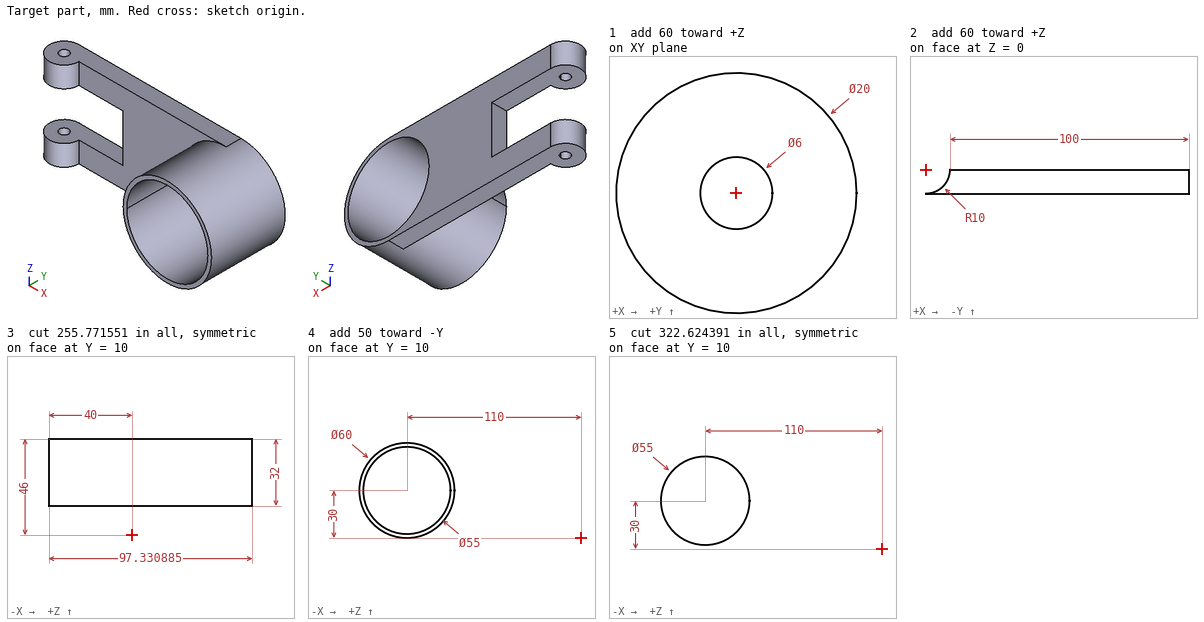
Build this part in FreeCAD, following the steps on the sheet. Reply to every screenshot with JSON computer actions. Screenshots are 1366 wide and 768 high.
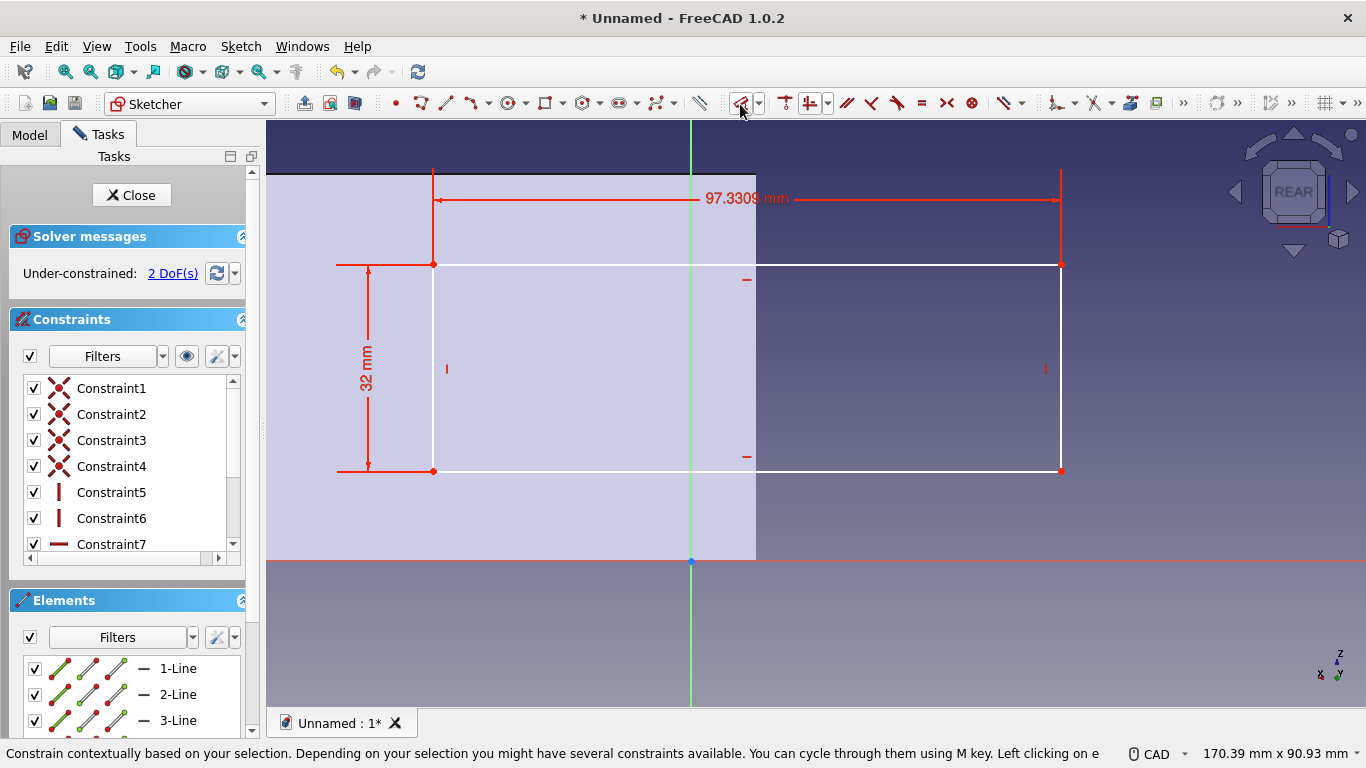
{"action": "left_click", "coordinate": [433, 265]}
{"action": "left_click", "coordinate": [562, 595]}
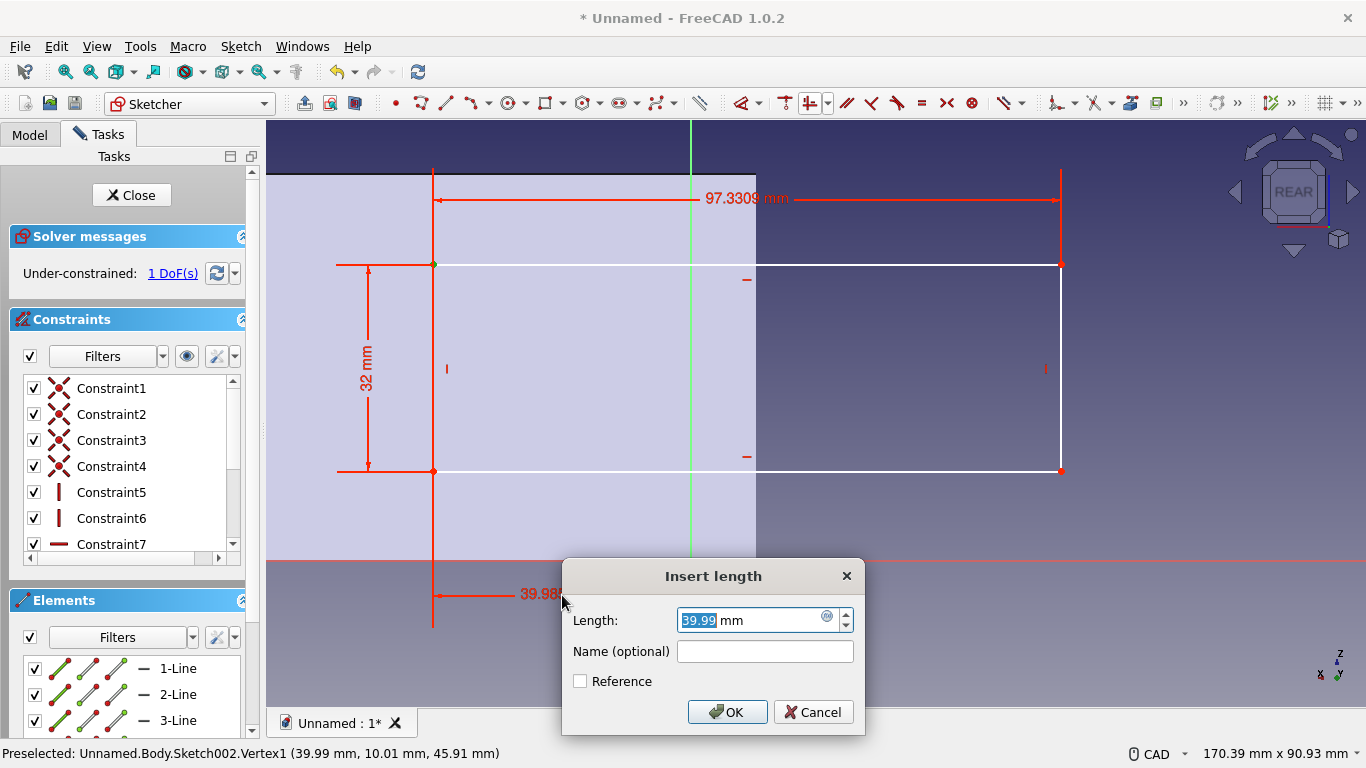
{"action": "type", "text": "40"}
{"action": "key", "text": "Return"}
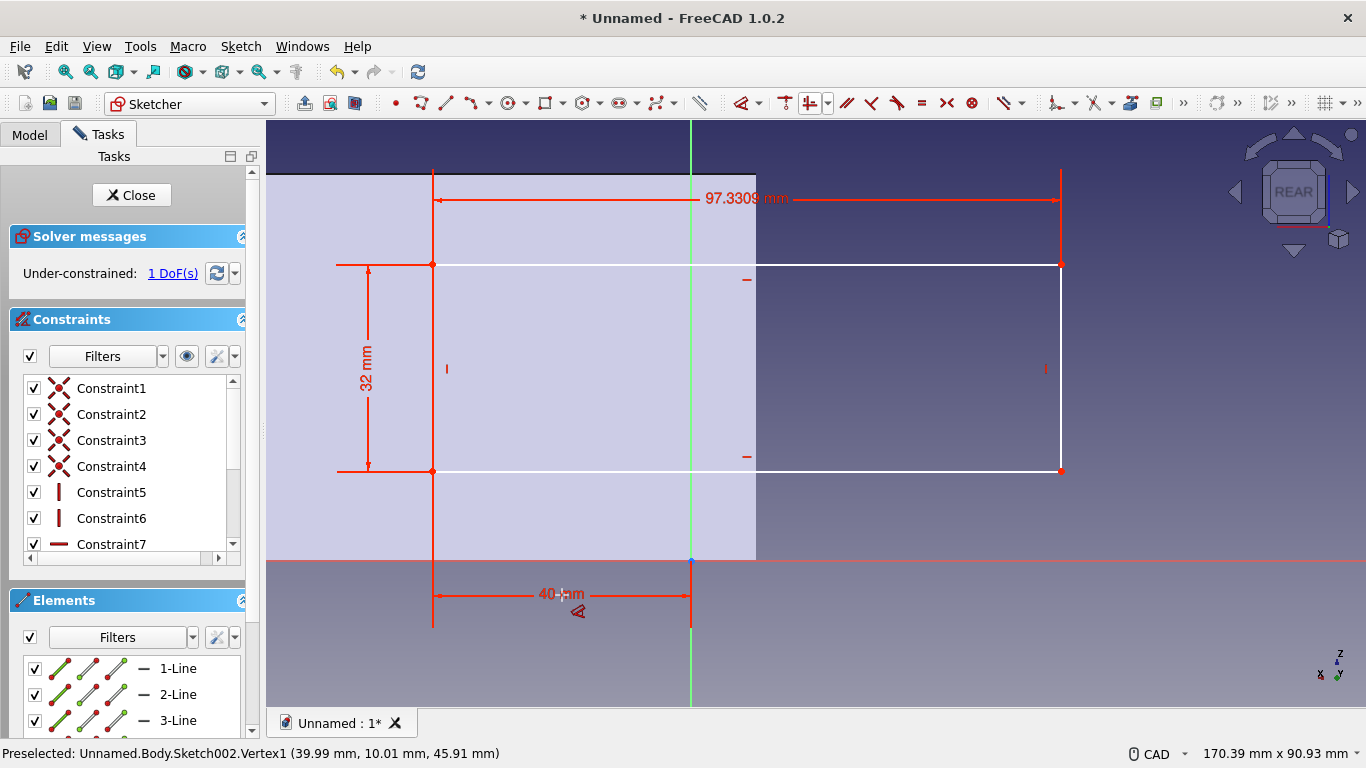
{"action": "left_click", "coordinate": [433, 265]}
{"action": "left_click", "coordinate": [399, 413]}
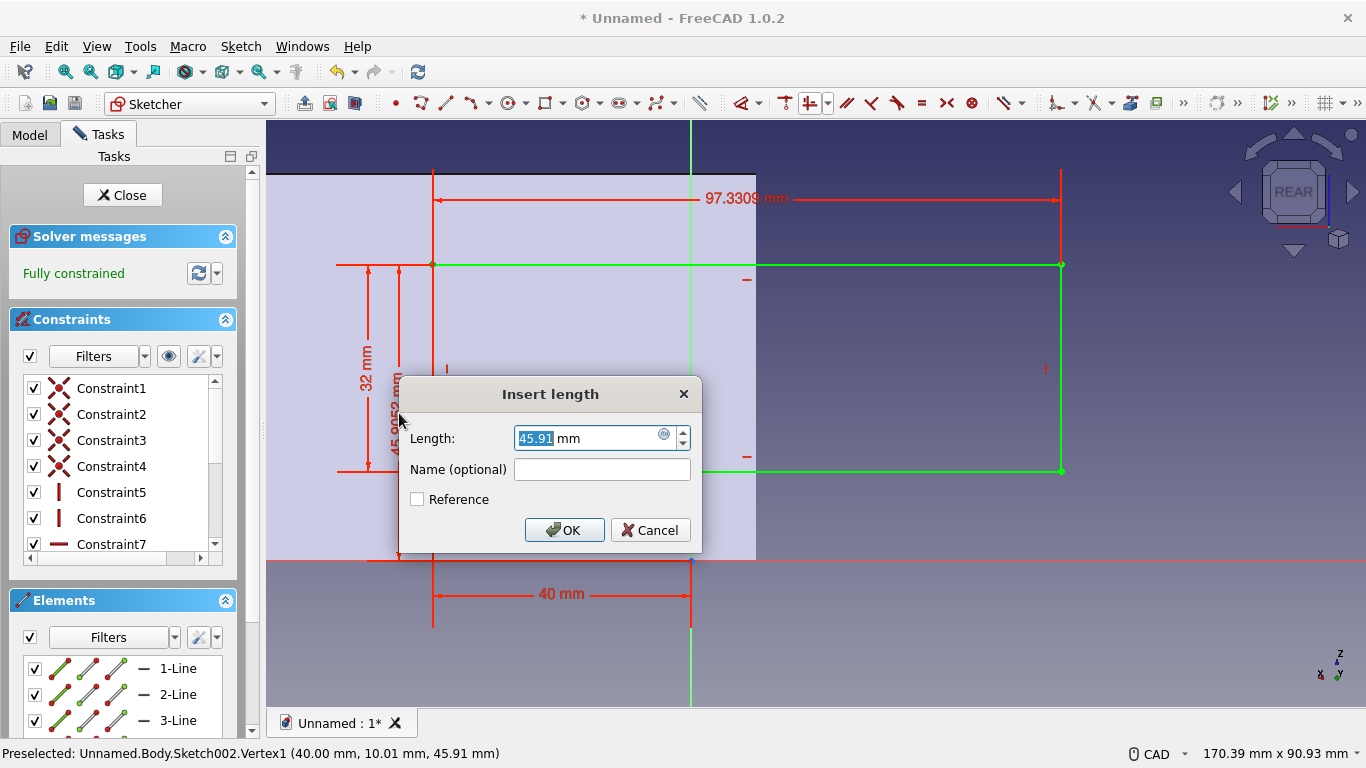
{"action": "type", "text": "46"}
{"action": "key", "text": "Return"}
{"action": "key", "text": "Escape"}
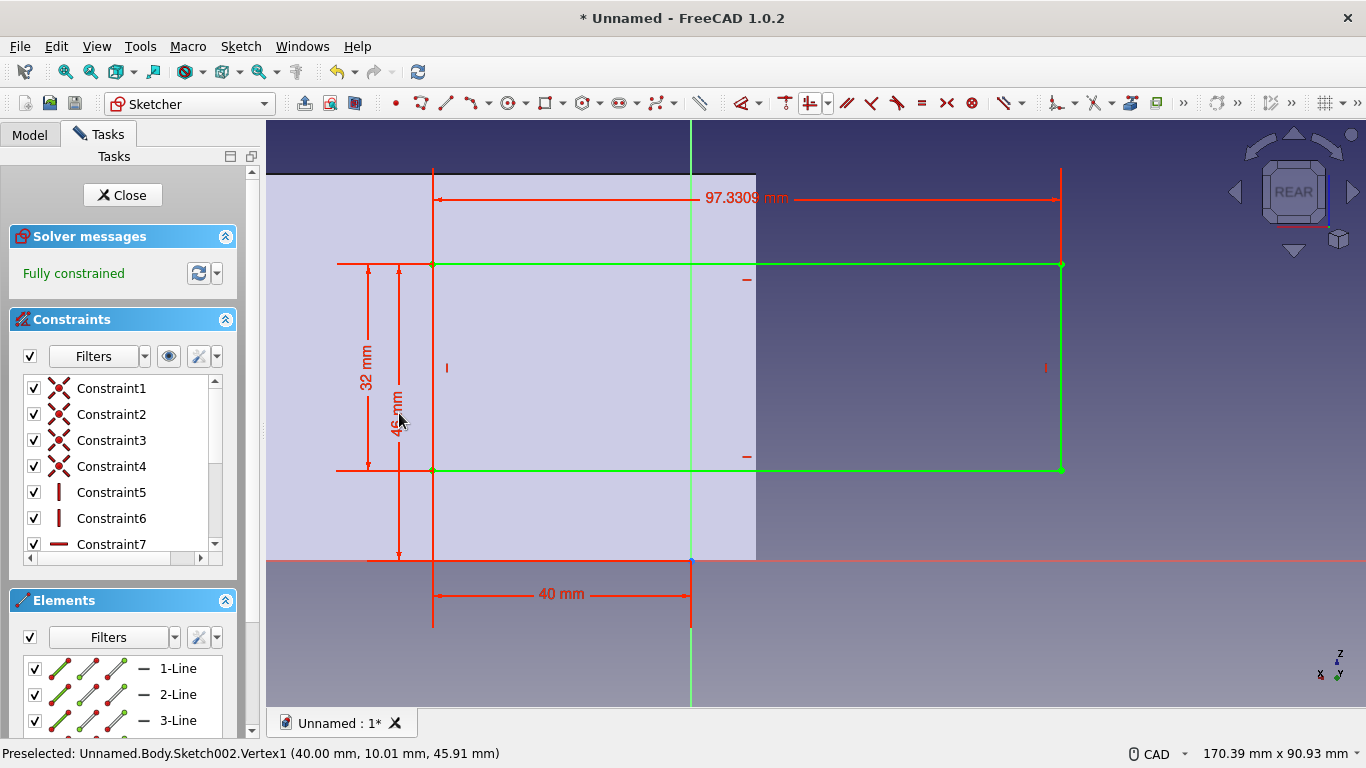
{"action": "left_click", "coordinate": [123, 195]}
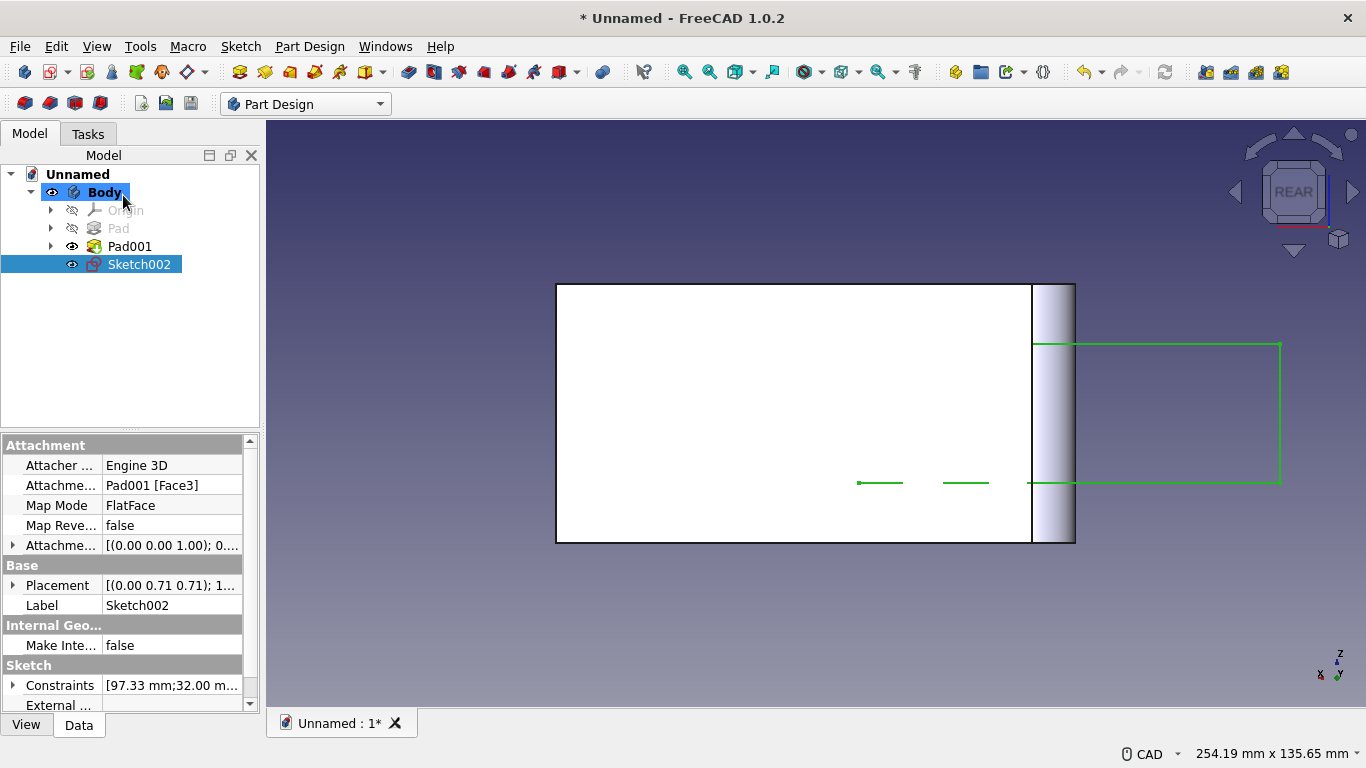
{"action": "left_click", "coordinate": [409, 72]}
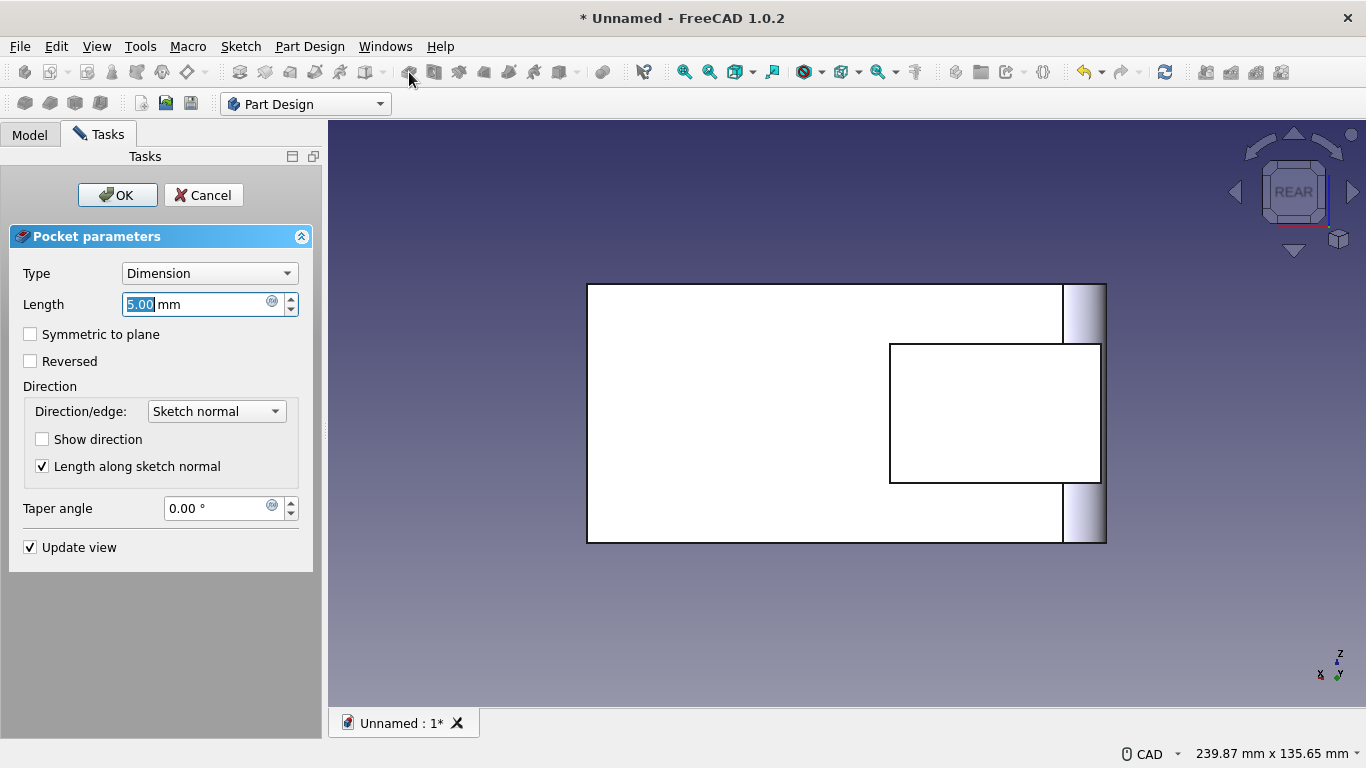
{"action": "type", "text": "255.771551"}
{"action": "key", "text": "Tab"}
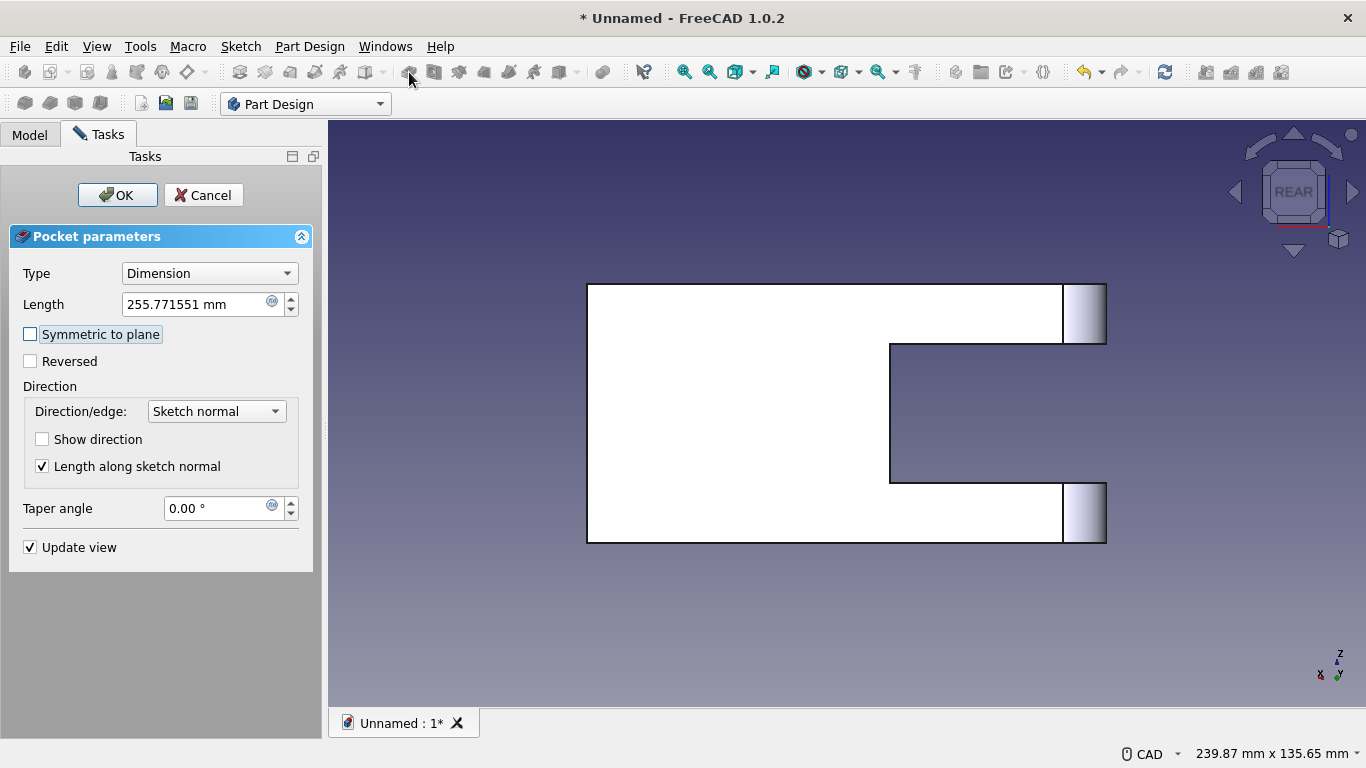
{"action": "left_click", "coordinate": [31, 334]}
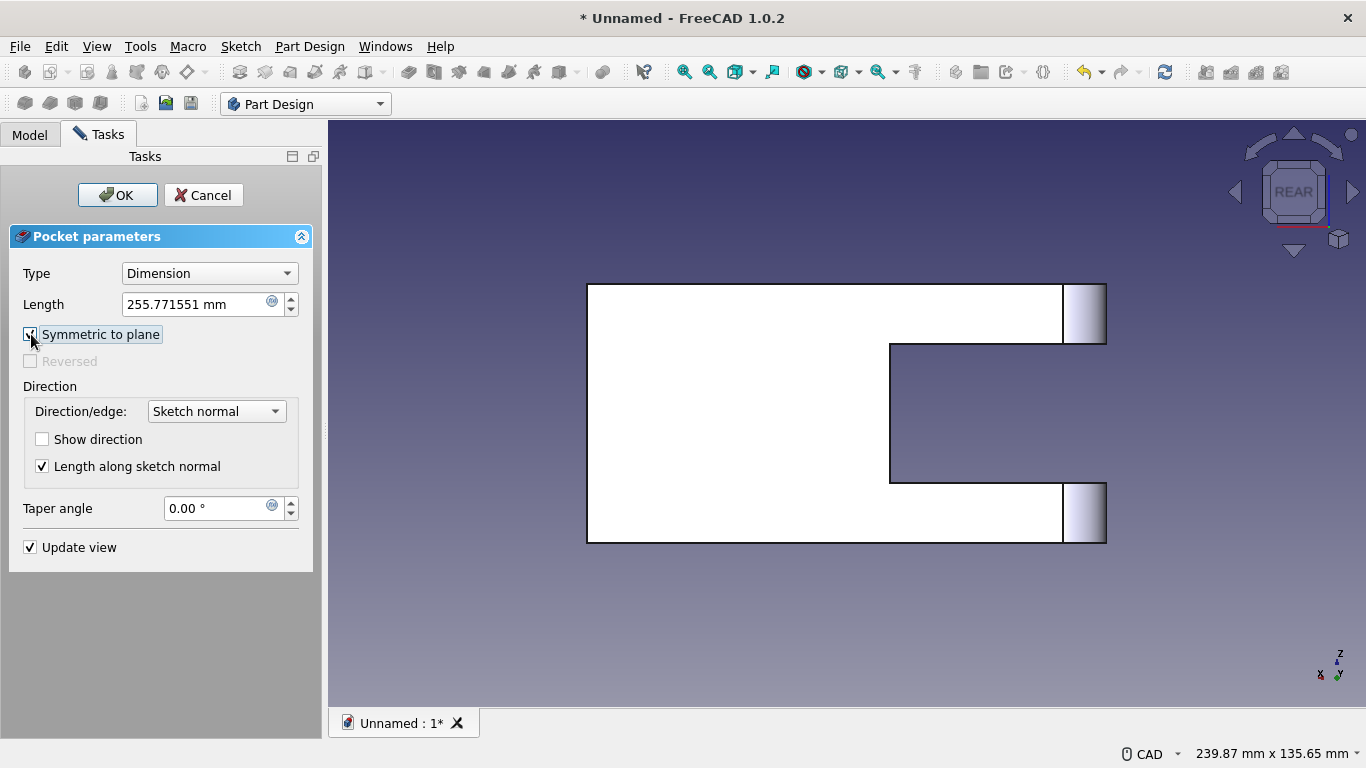
{"action": "left_click", "coordinate": [118, 195]}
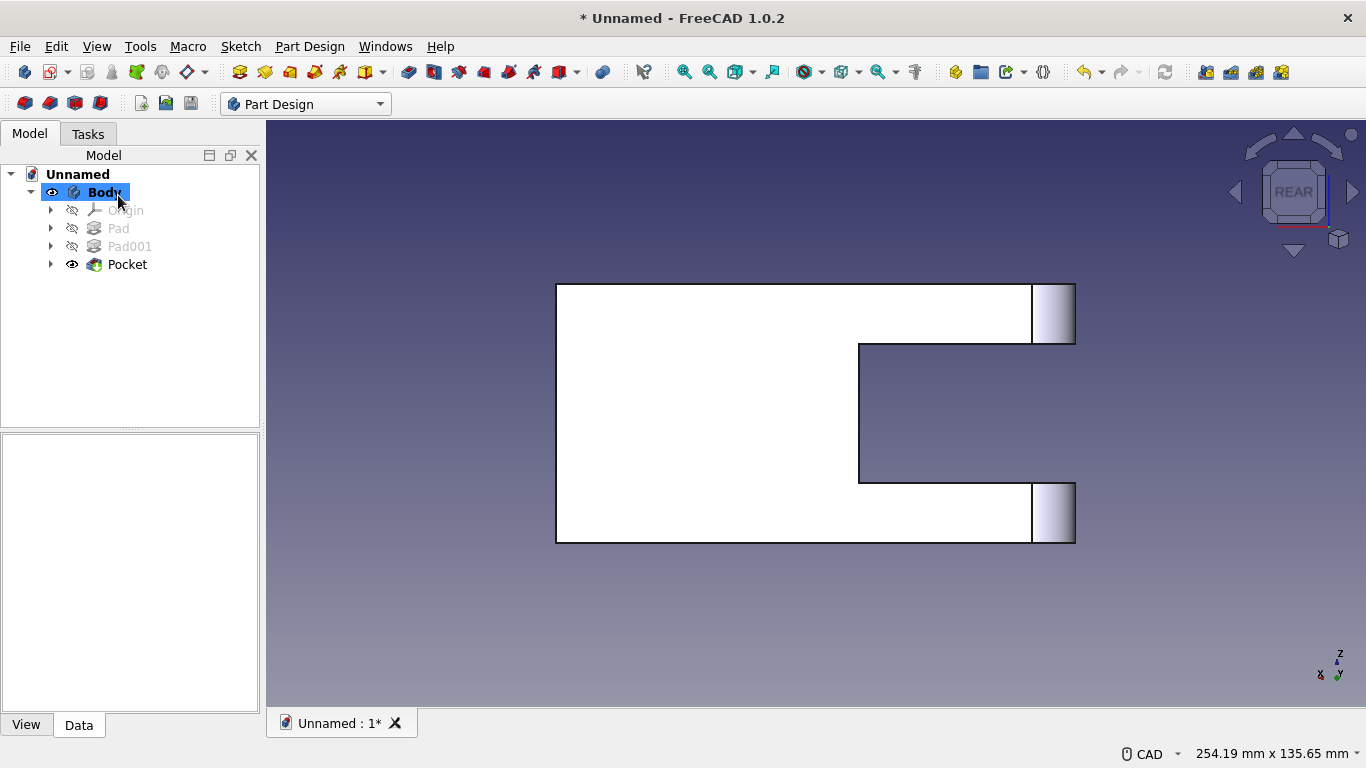
{"action": "left_click", "coordinate": [726, 412]}